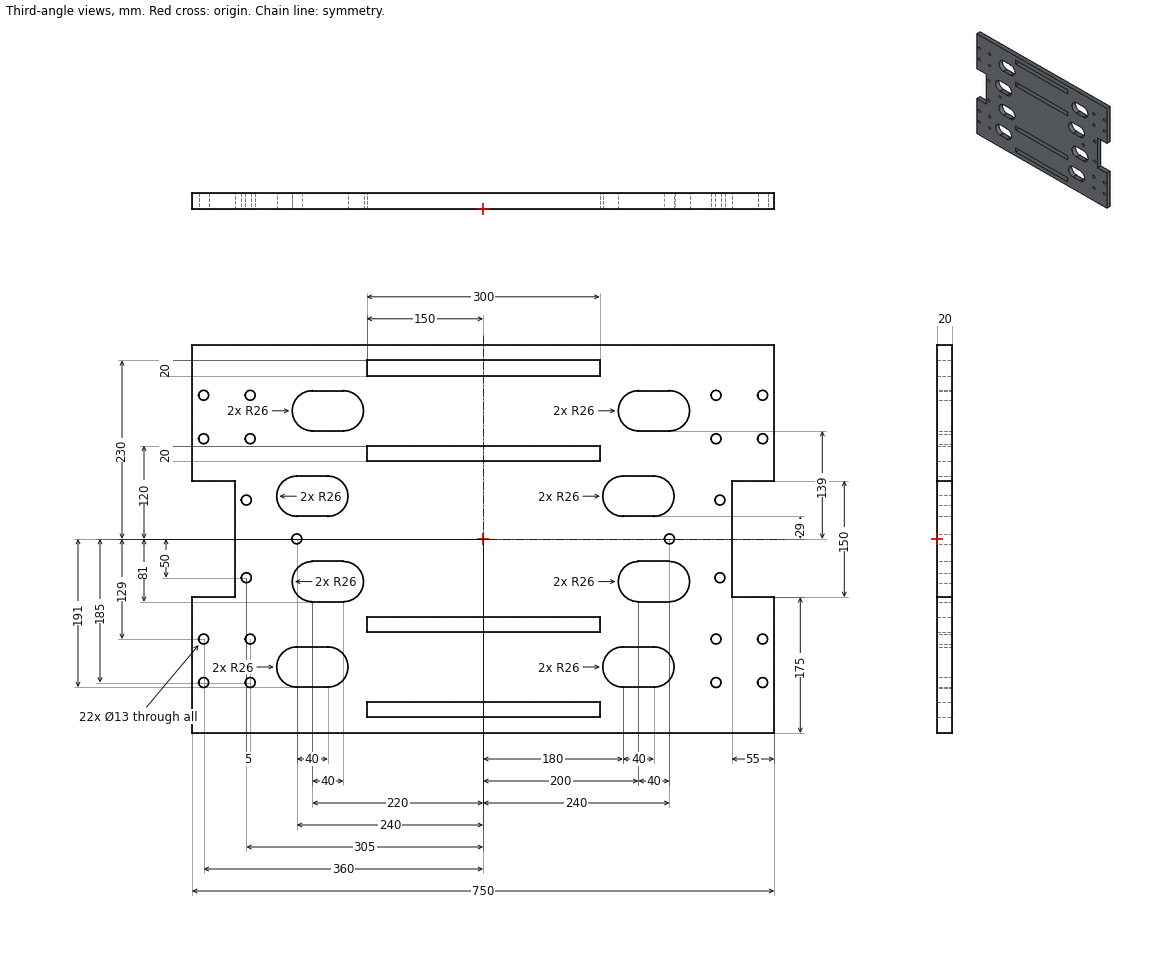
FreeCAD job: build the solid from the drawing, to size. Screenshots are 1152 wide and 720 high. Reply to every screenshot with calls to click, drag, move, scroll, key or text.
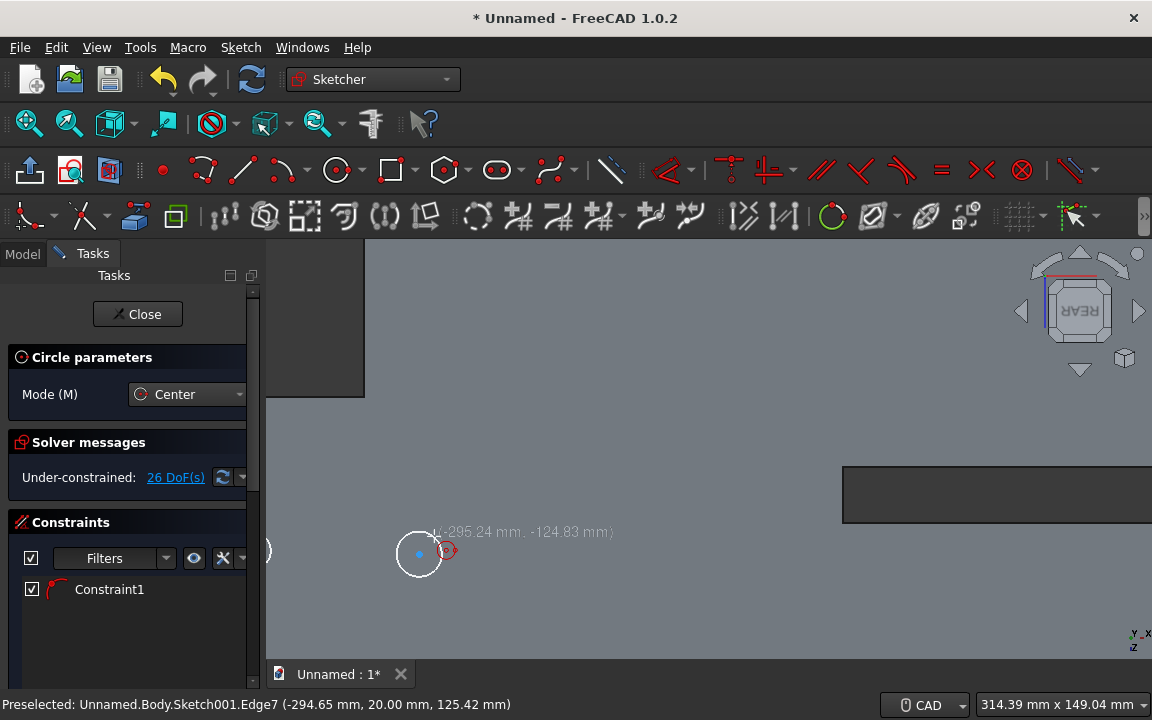
scroll(436, 535, down, 7)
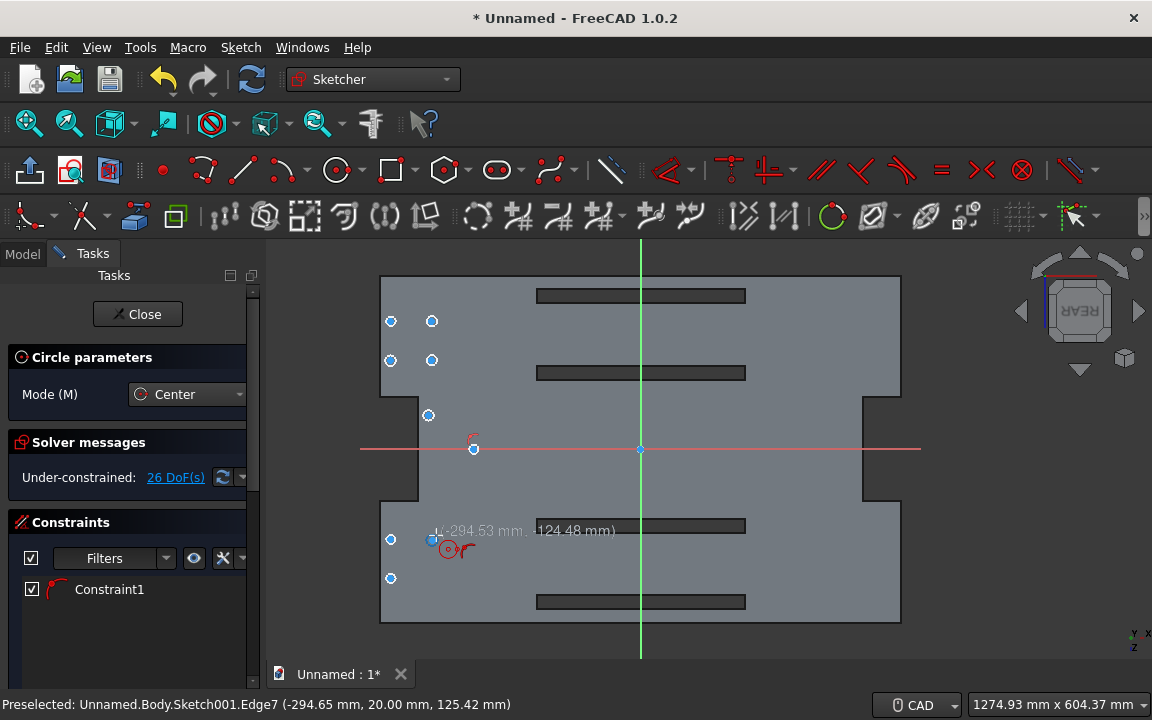
scroll(432, 578, up, 9)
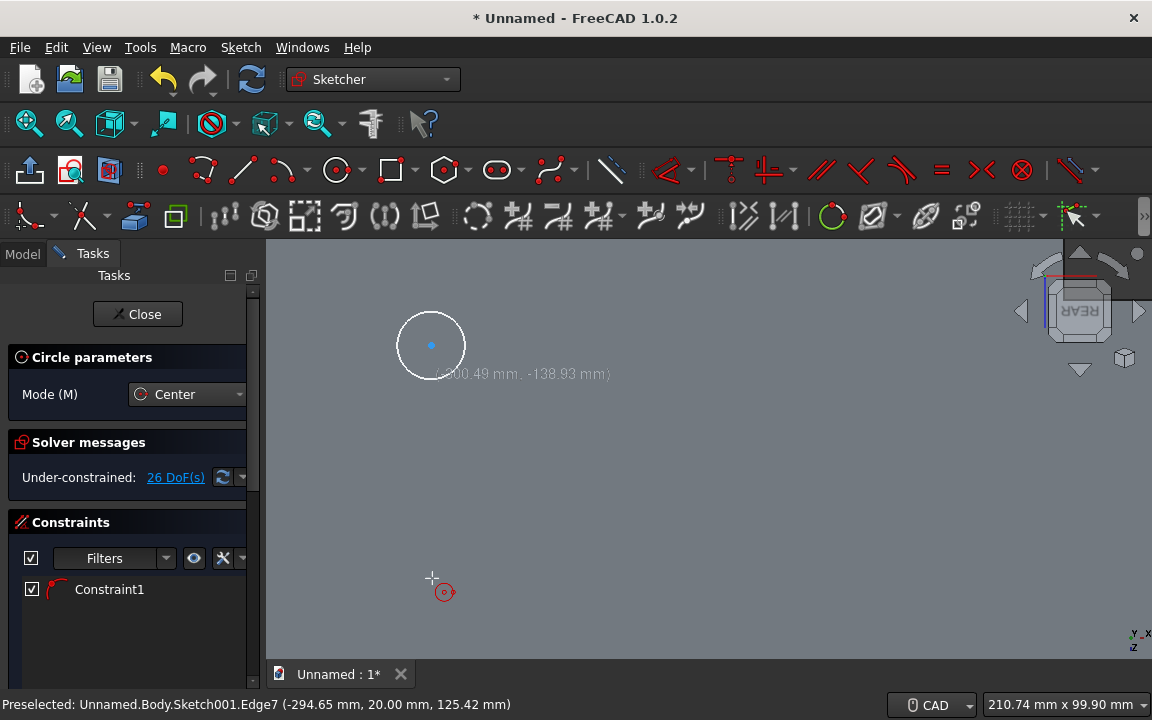
scroll(432, 578, down, 9)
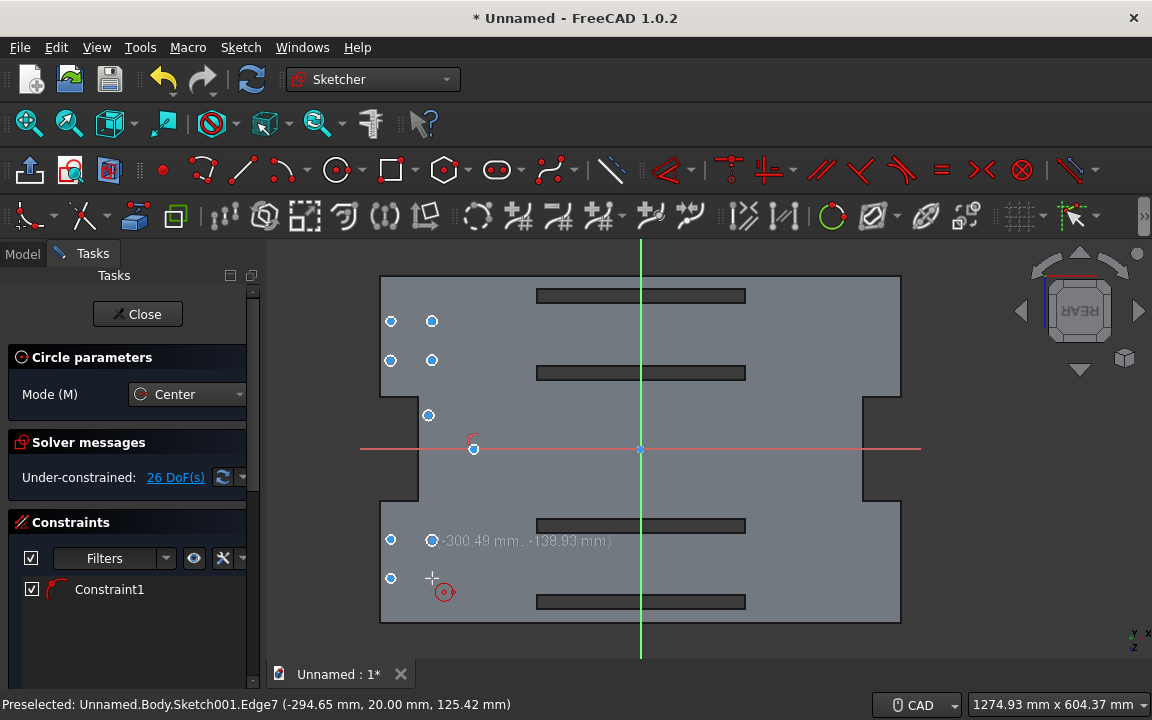
click(432, 578)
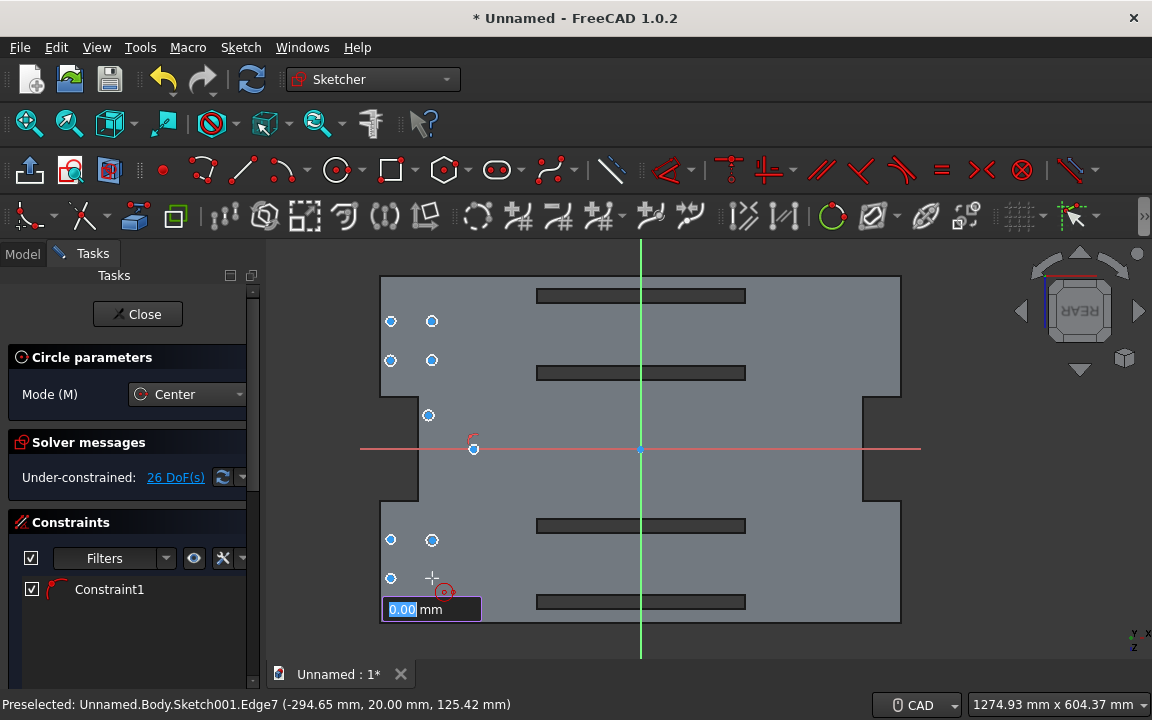
scroll(436, 575, up, 7)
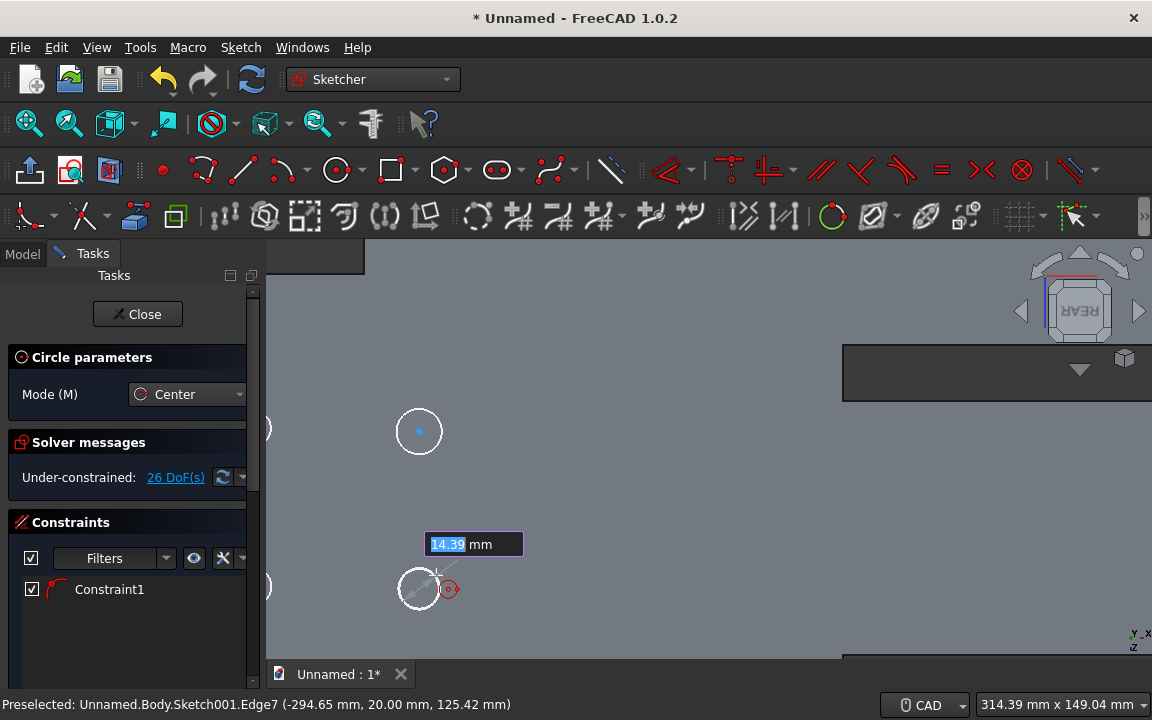
click(434, 571)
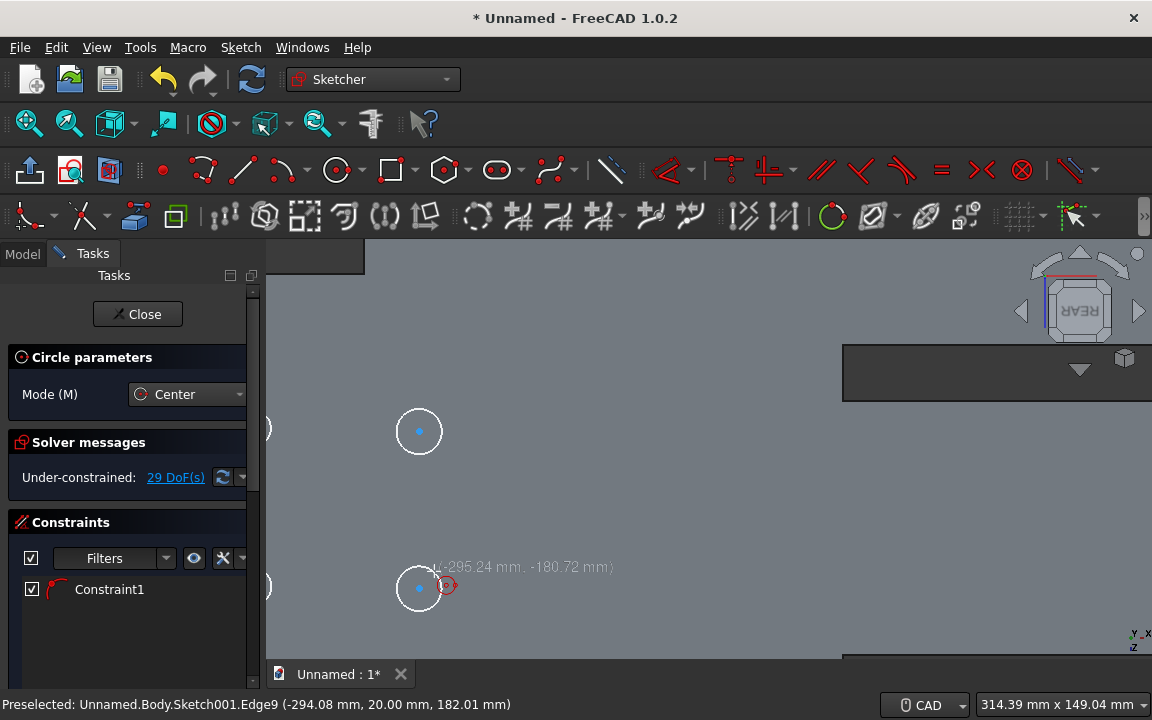
scroll(436, 575, down, 7)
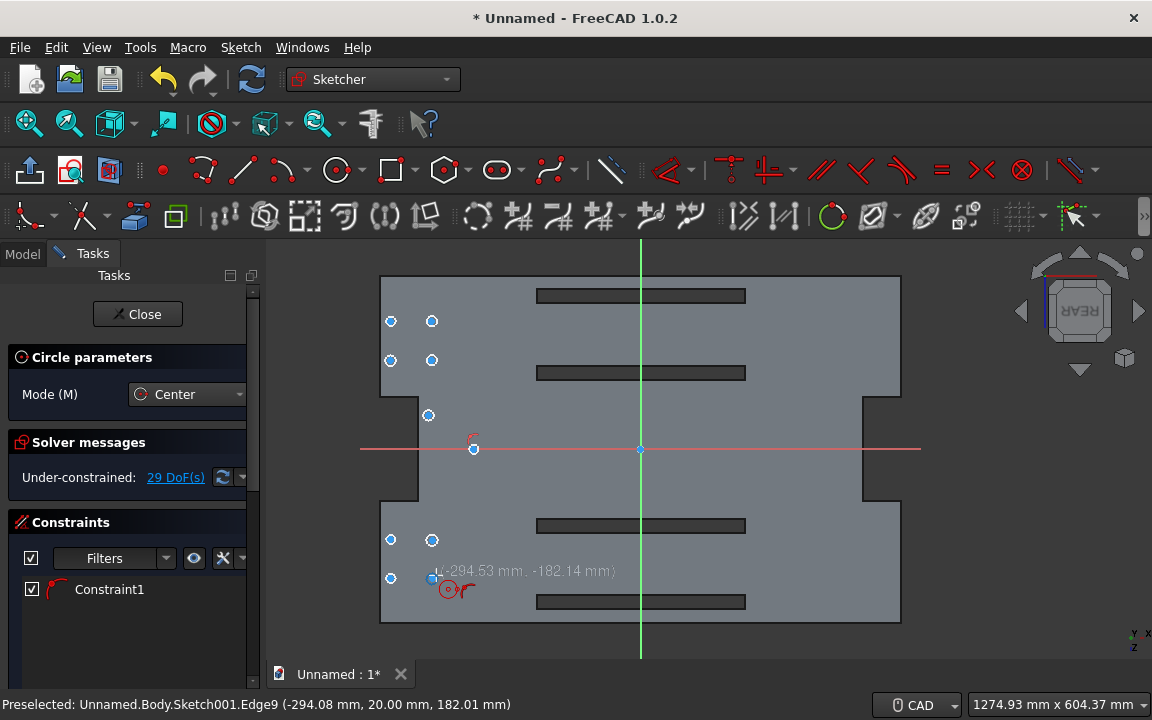
scroll(429, 484, up, 9)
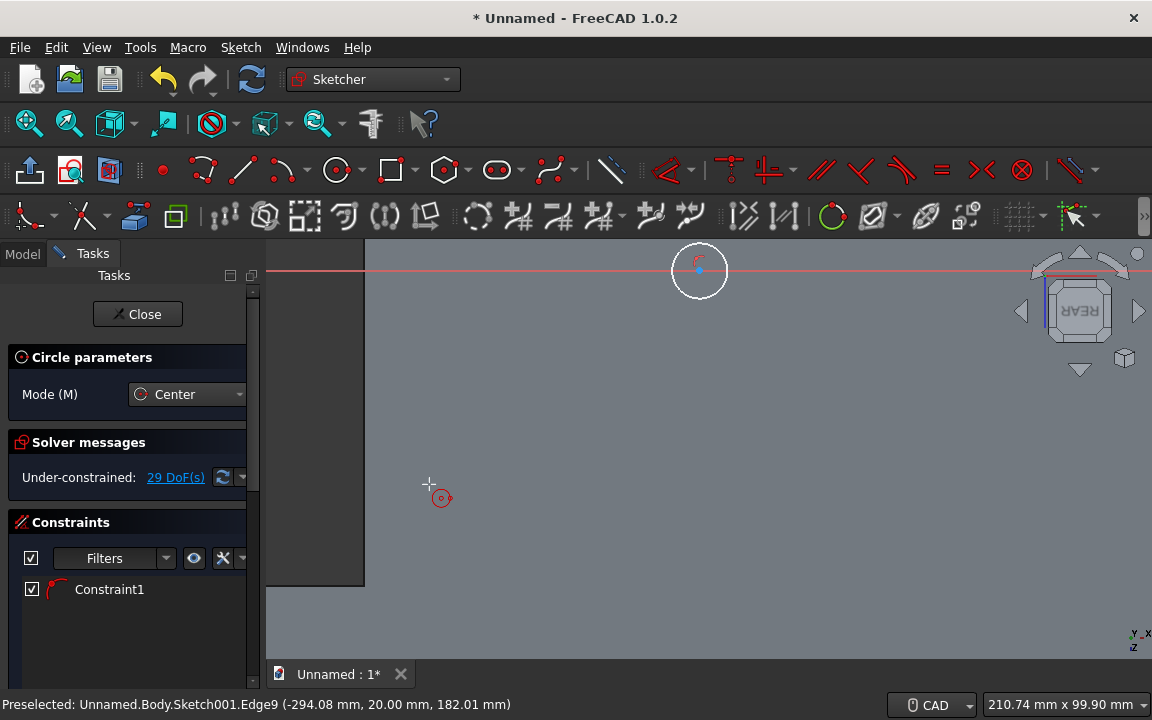
scroll(429, 484, down, 9)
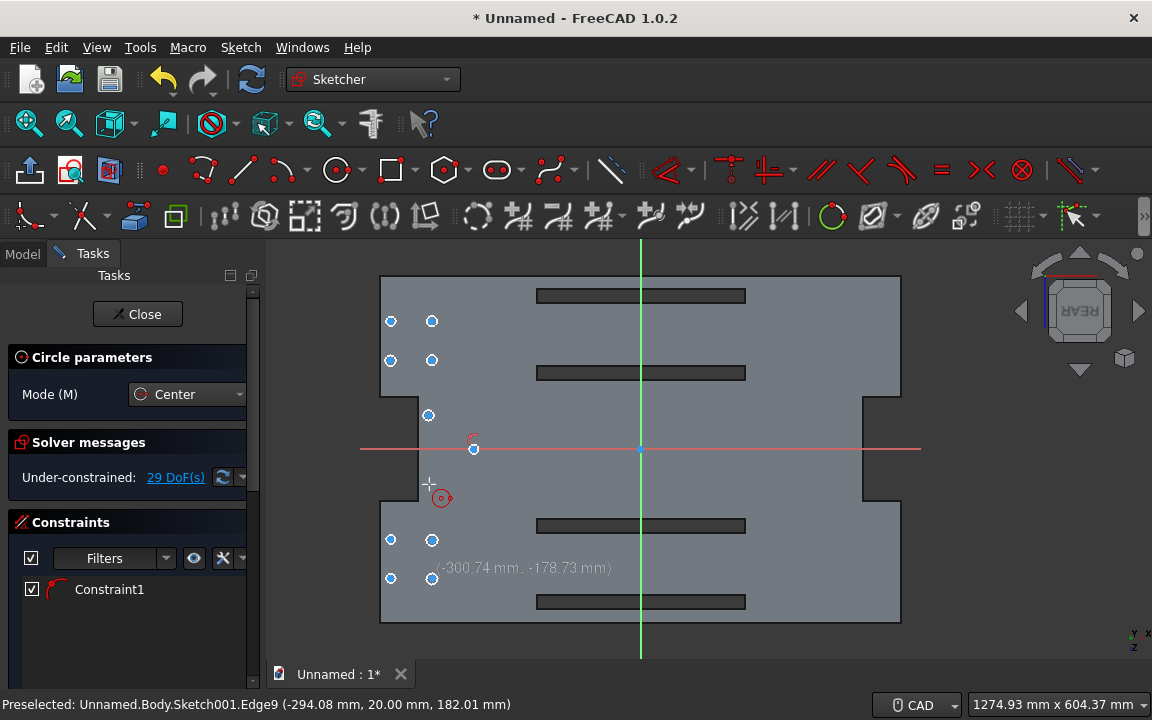
click(429, 484)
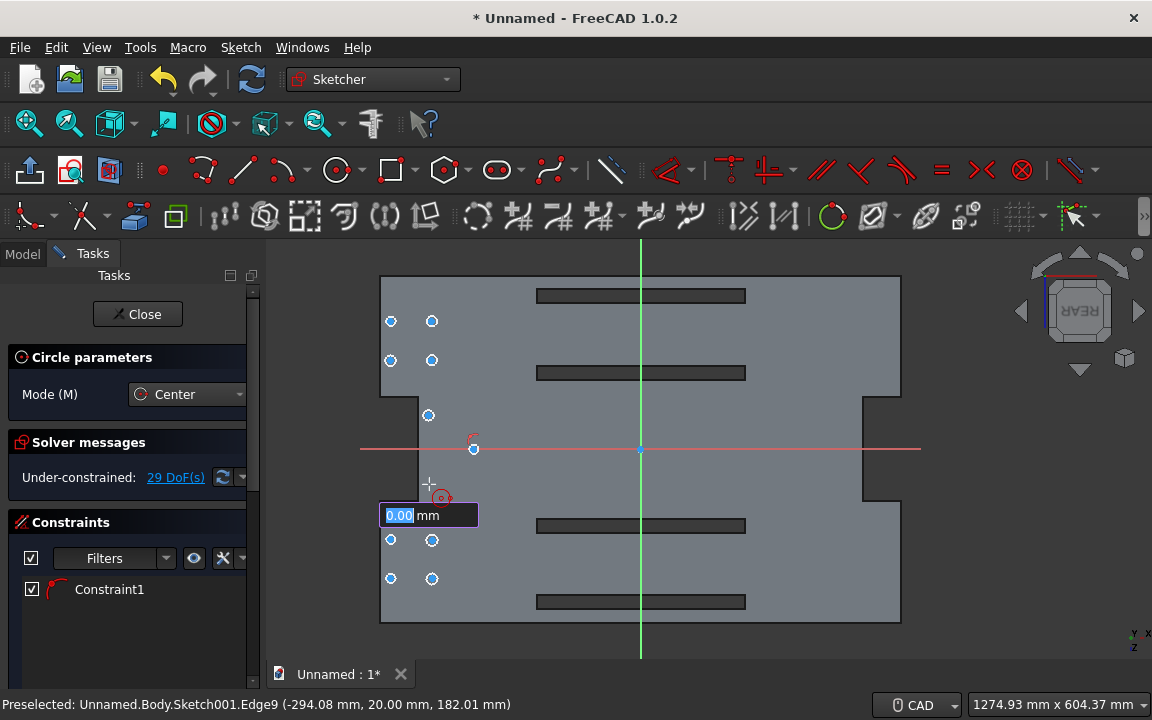
scroll(432, 481, up, 7)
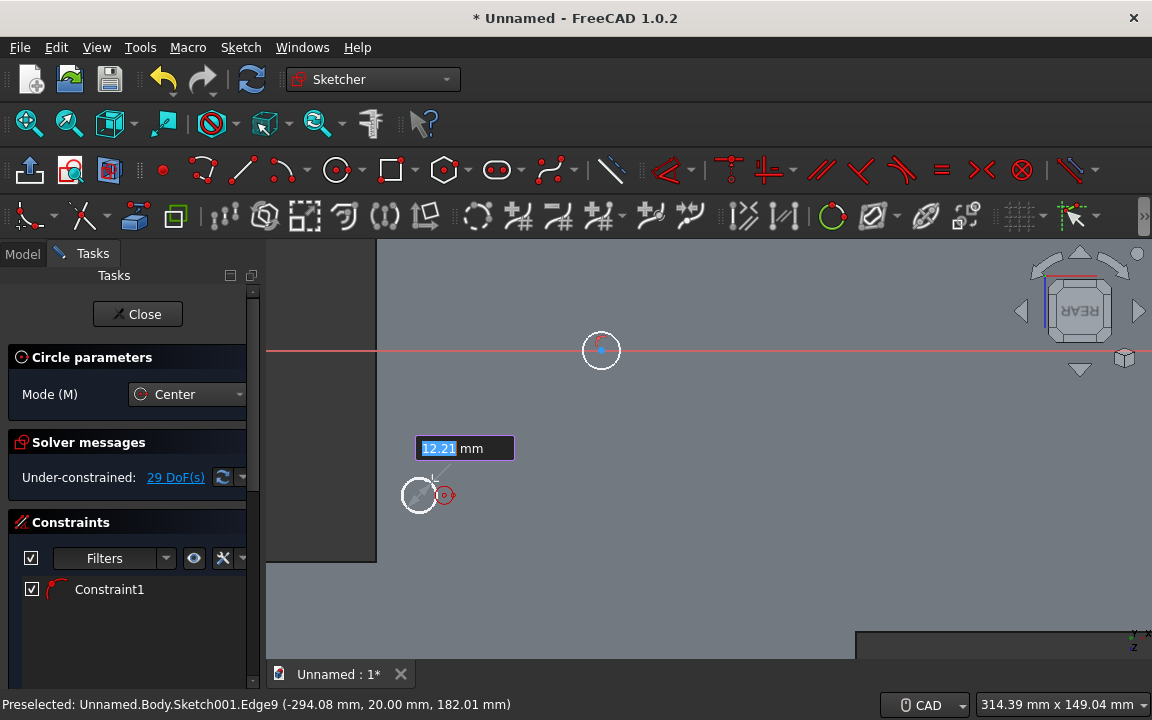
click(432, 479)